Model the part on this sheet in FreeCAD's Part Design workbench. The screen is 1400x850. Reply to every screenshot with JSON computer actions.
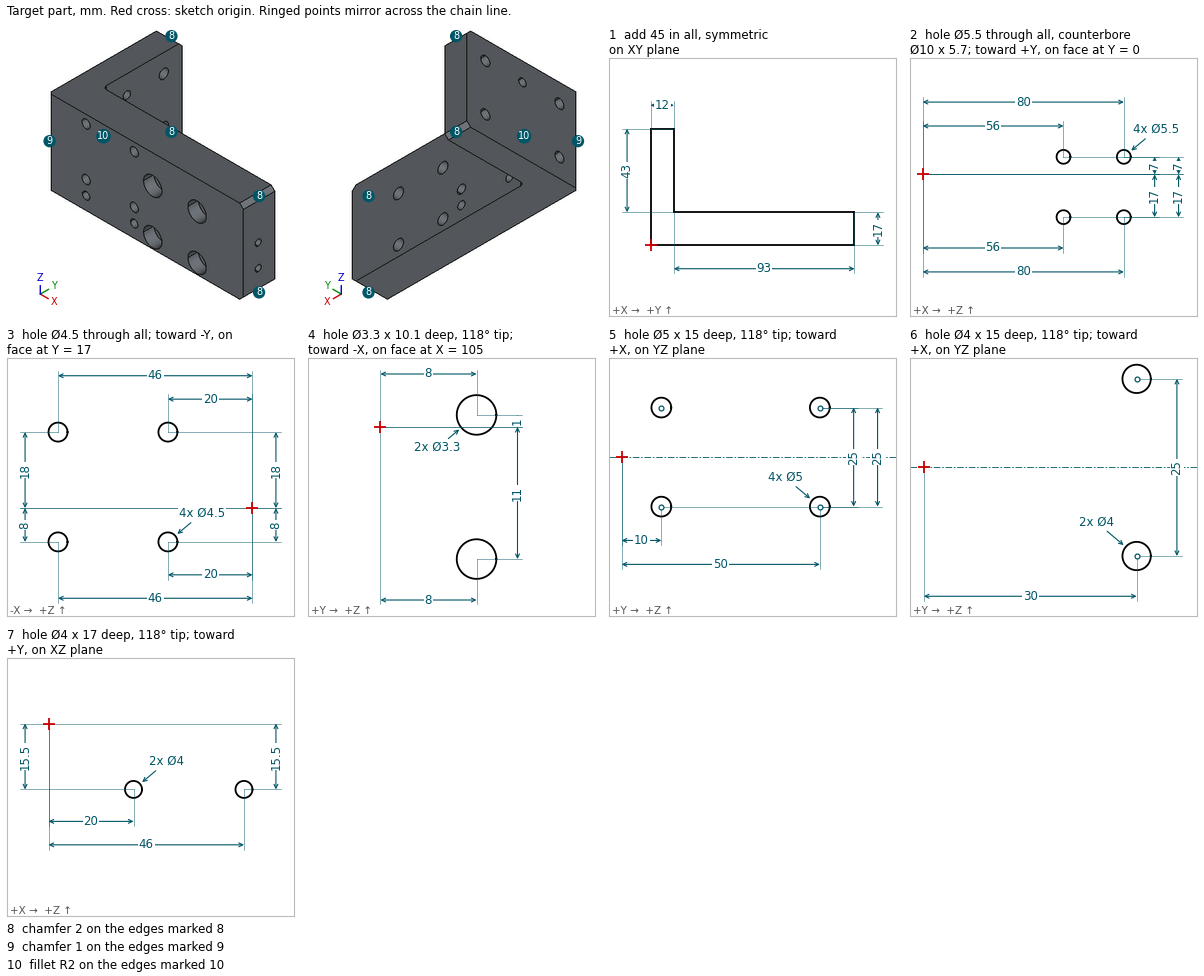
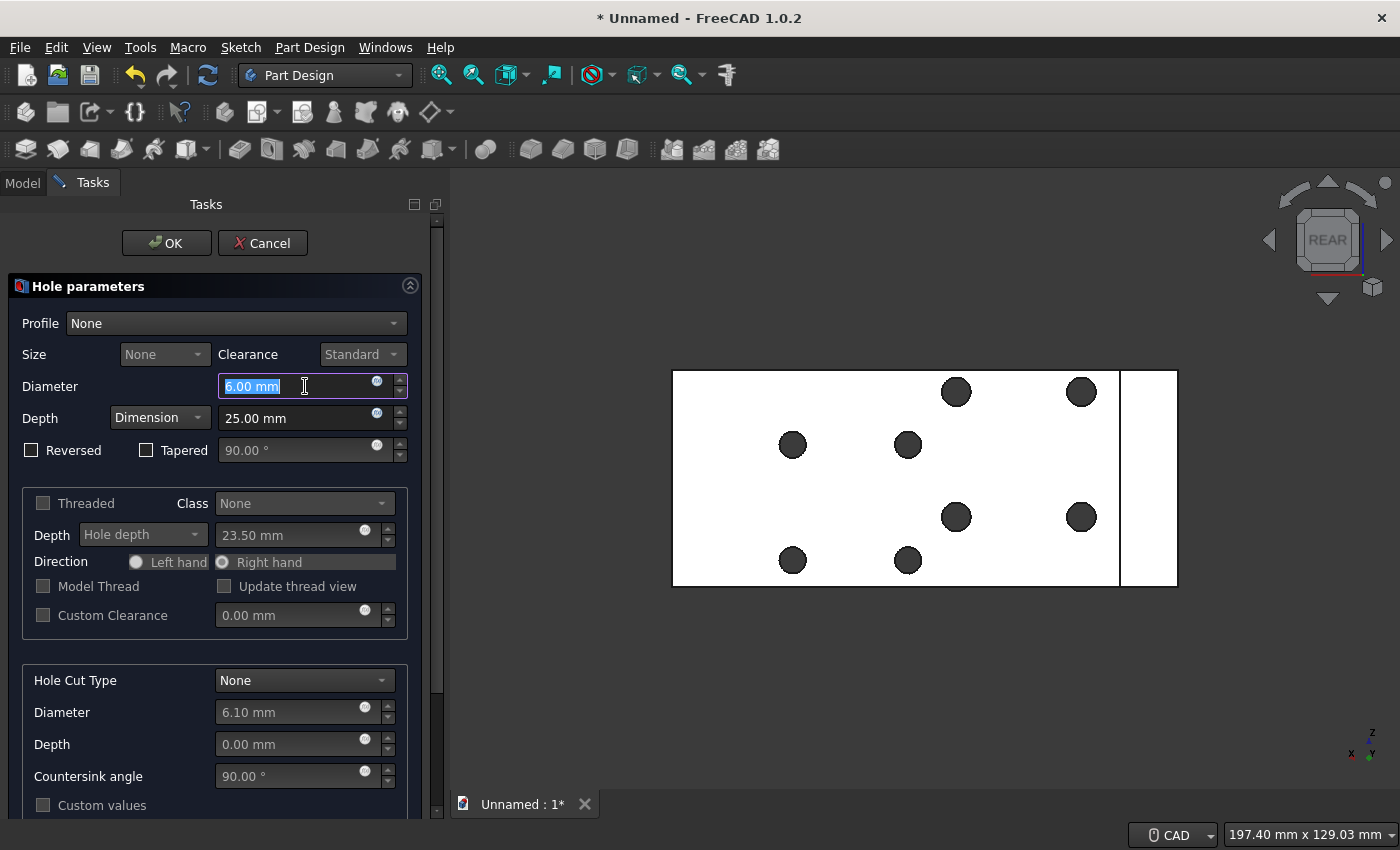
{"action": "type", "text": "4.5"}
{"action": "key", "text": "Tab"}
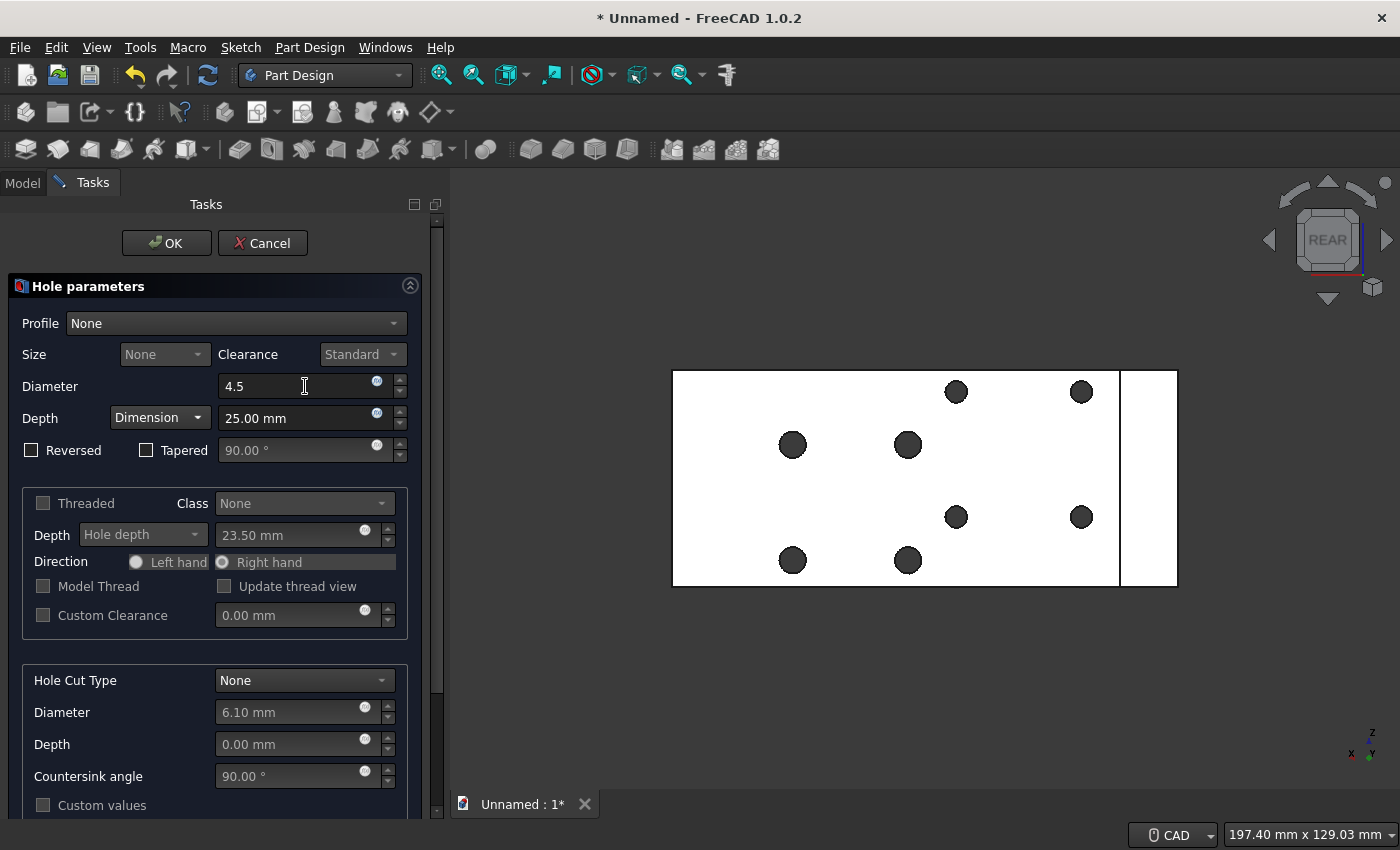
{"action": "left_click", "coordinate": [161, 418]}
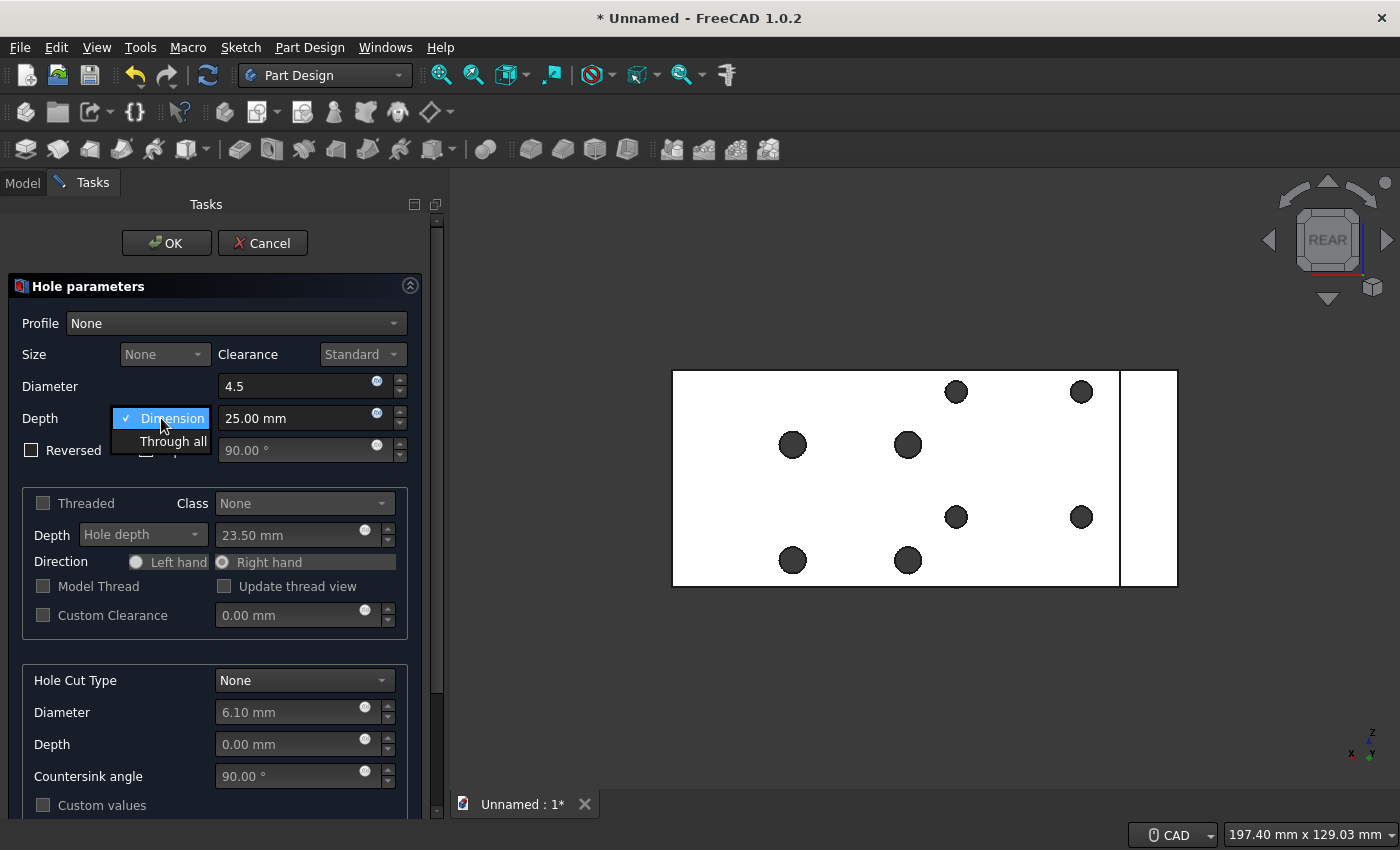
{"action": "left_click", "coordinate": [160, 442]}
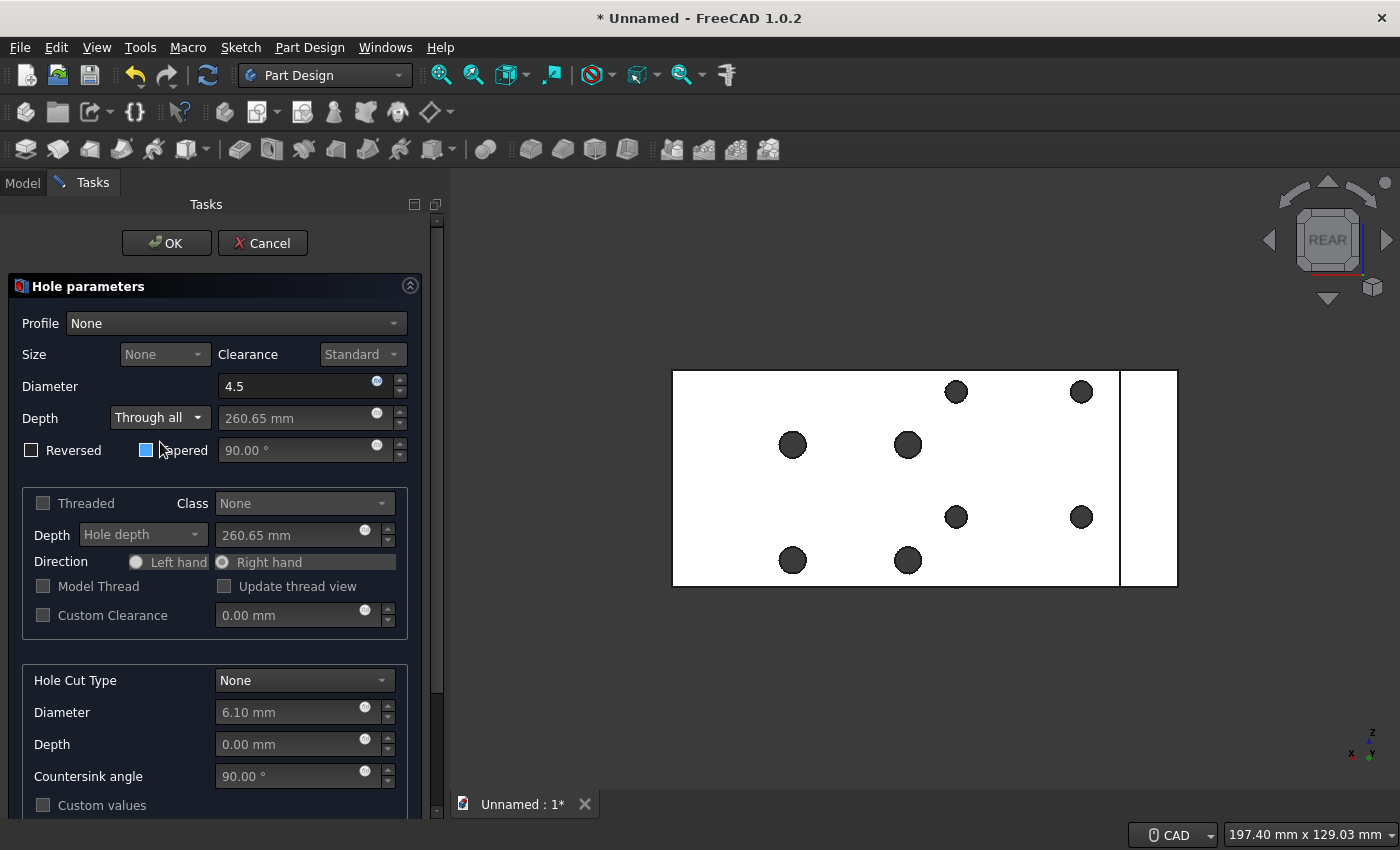
{"action": "left_click", "coordinate": [167, 243]}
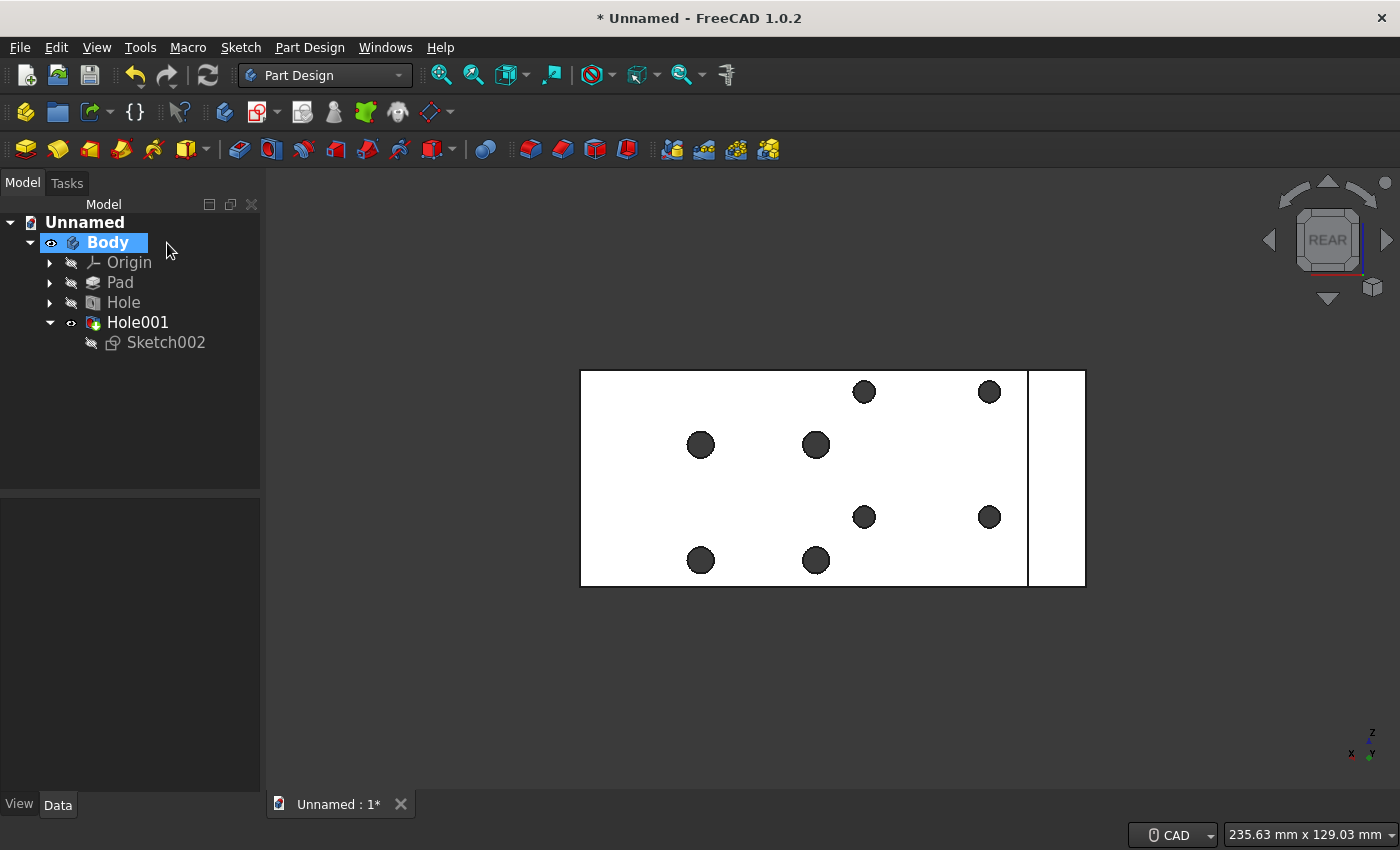
{"action": "key", "text": "v f"}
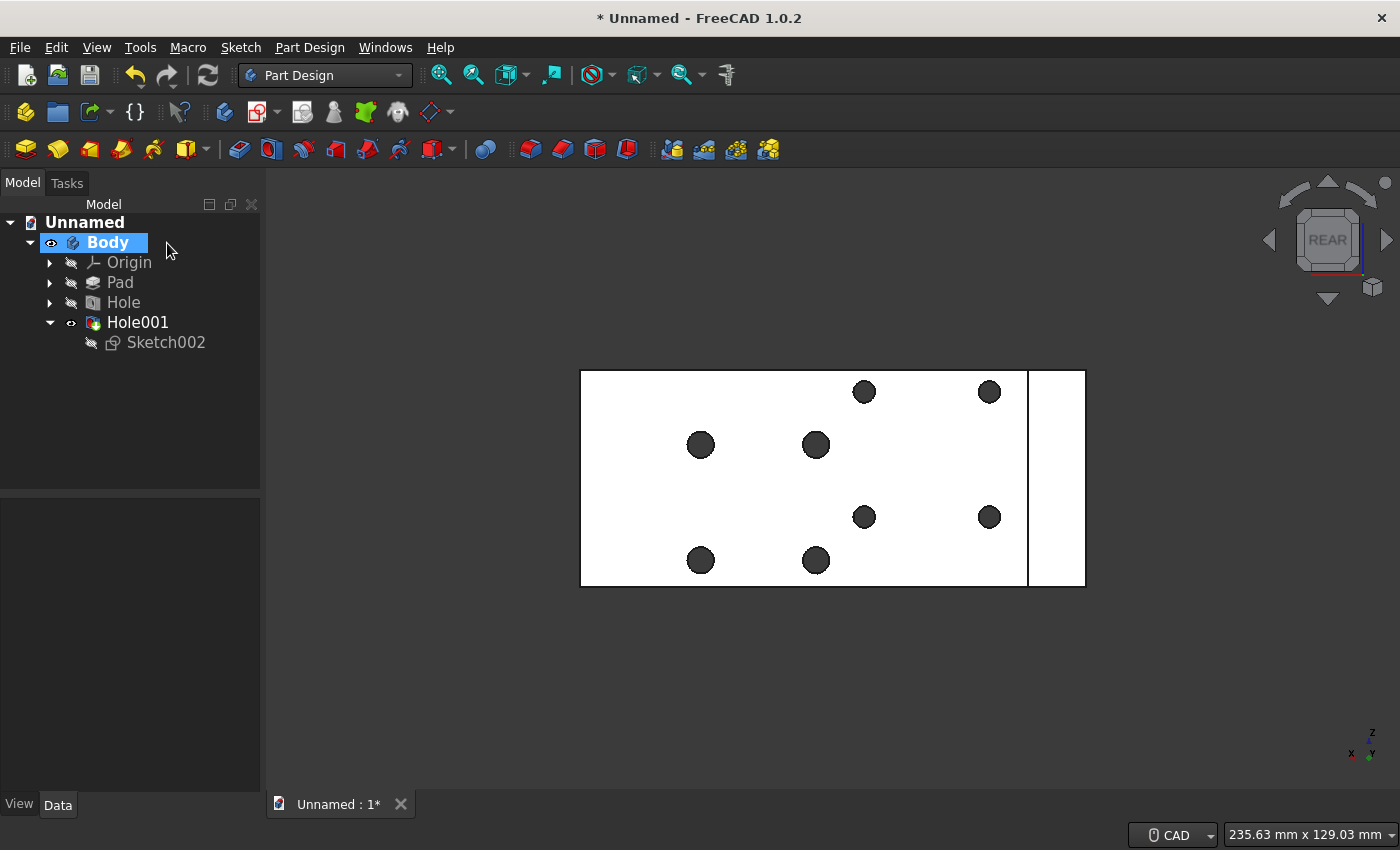
{"action": "key", "text": "0"}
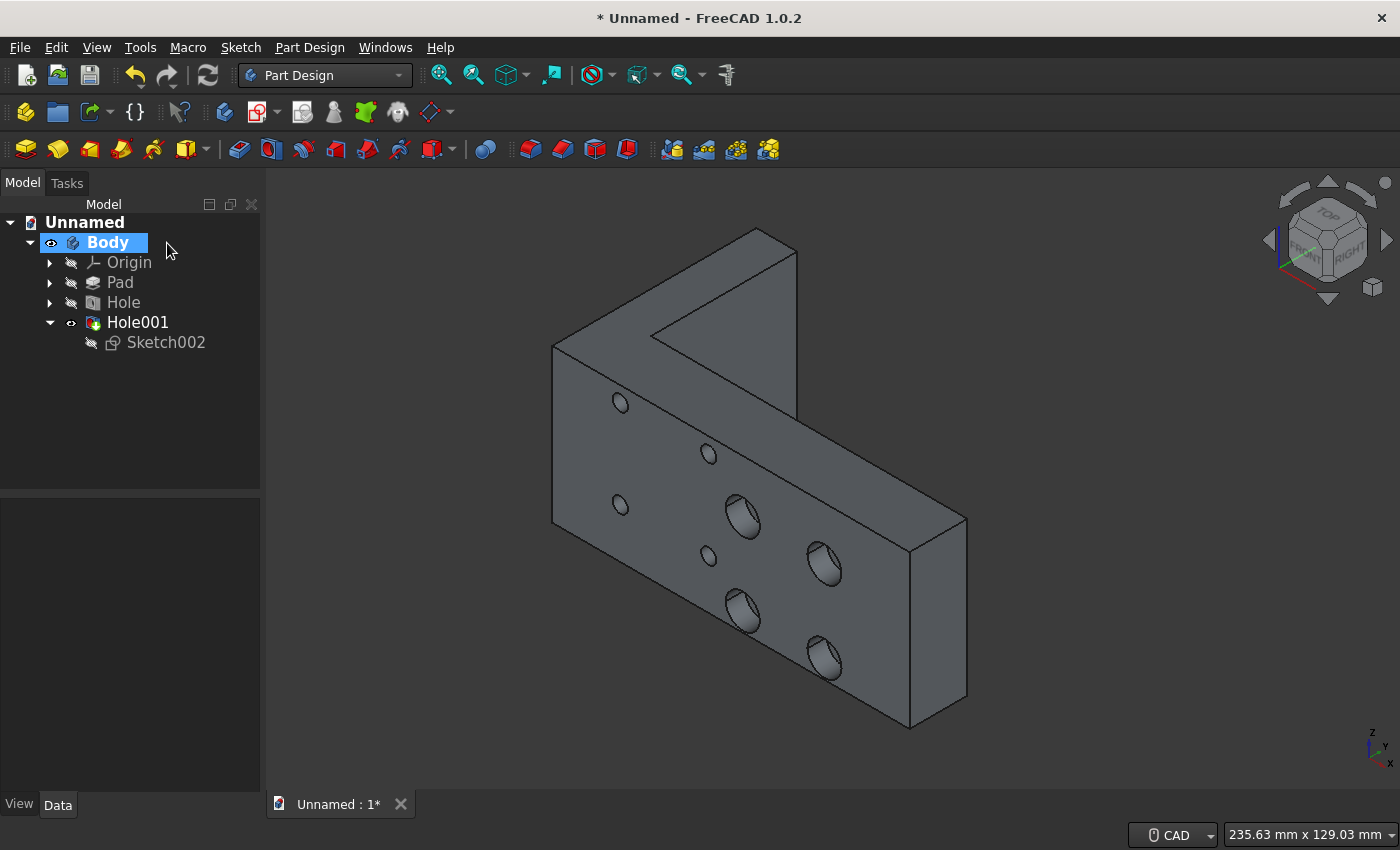
{"action": "left_click", "coordinate": [938, 572]}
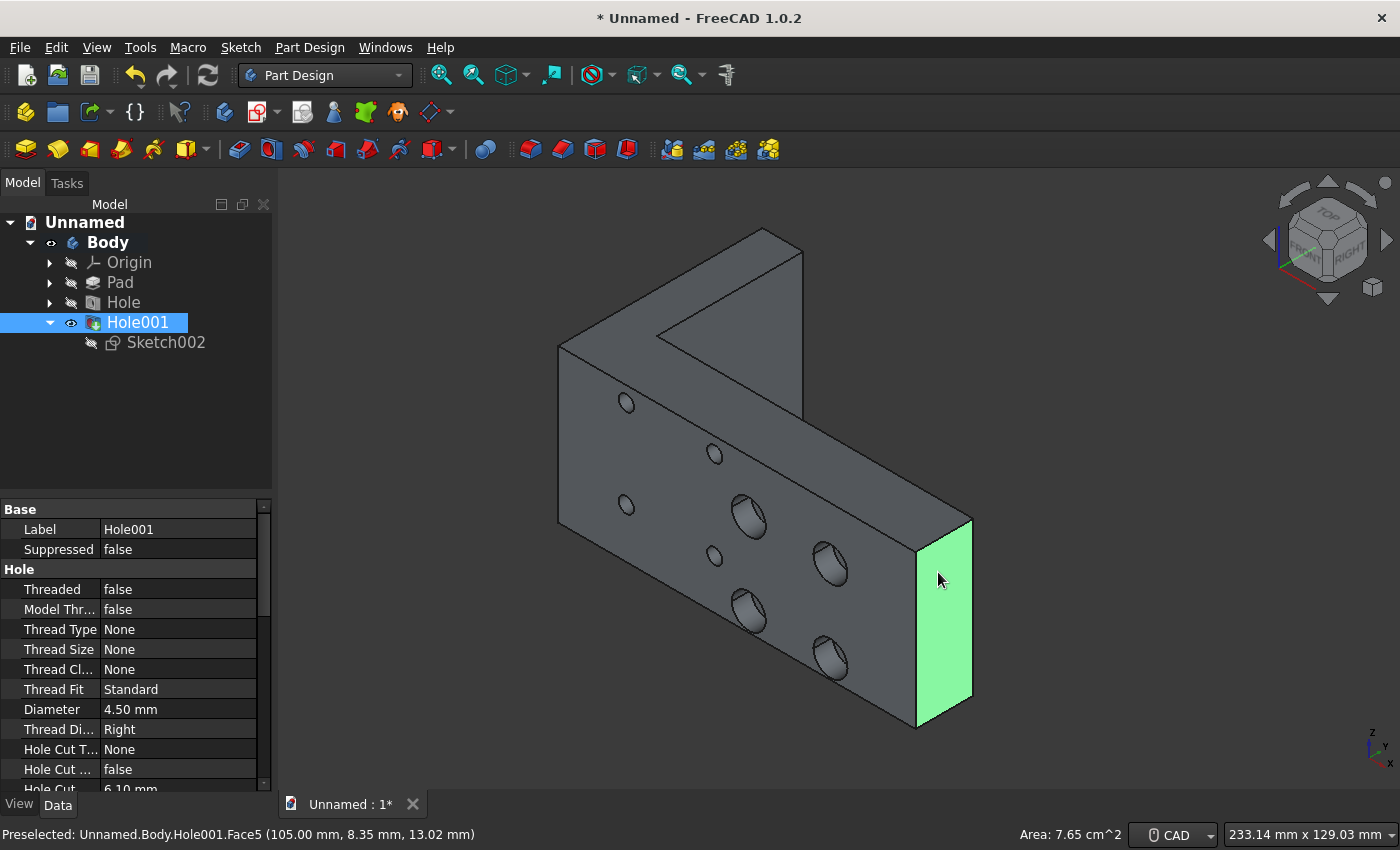
{"action": "left_click", "coordinate": [258, 112]}